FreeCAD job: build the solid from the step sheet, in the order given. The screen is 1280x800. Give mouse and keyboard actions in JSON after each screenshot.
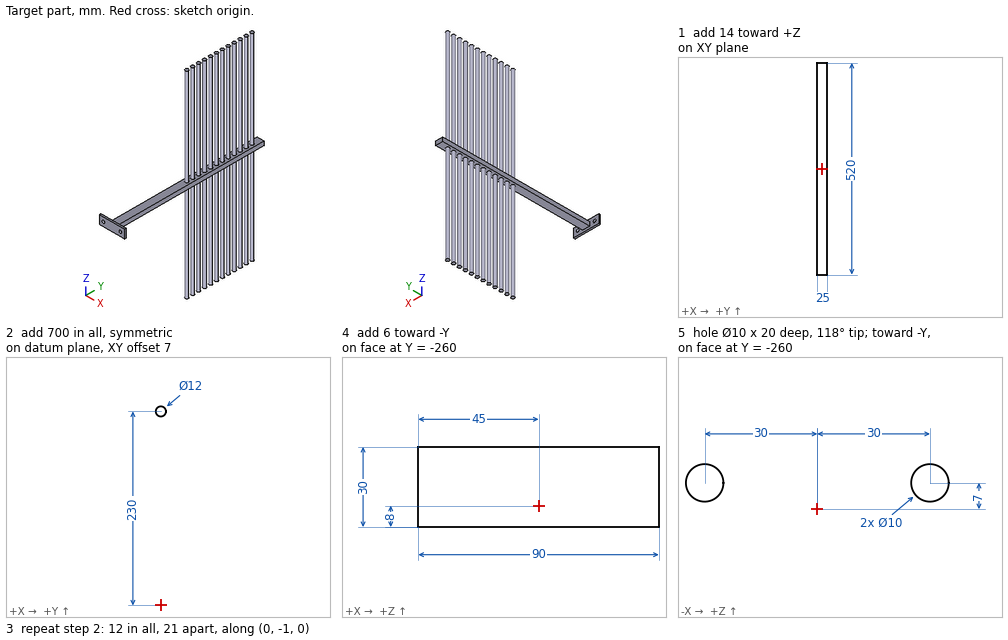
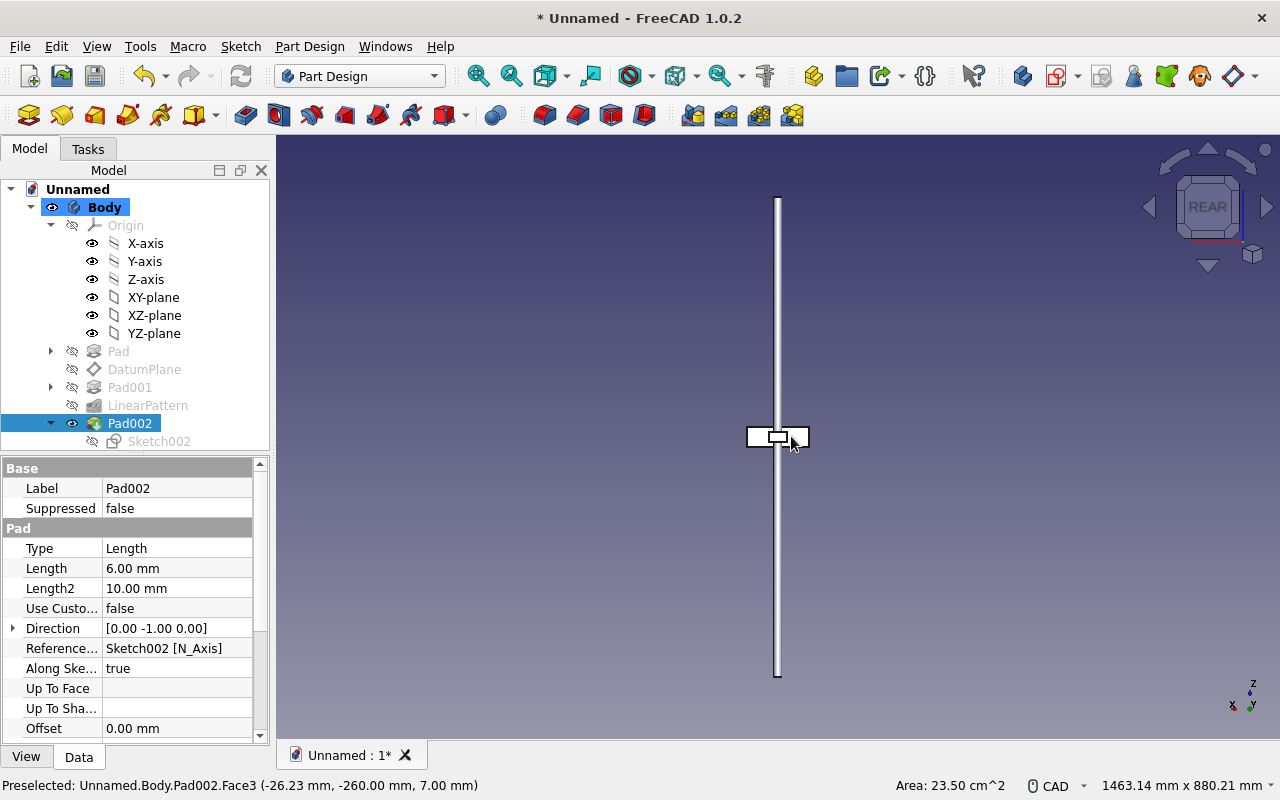
{"action": "left_click", "coordinate": [1056, 76]}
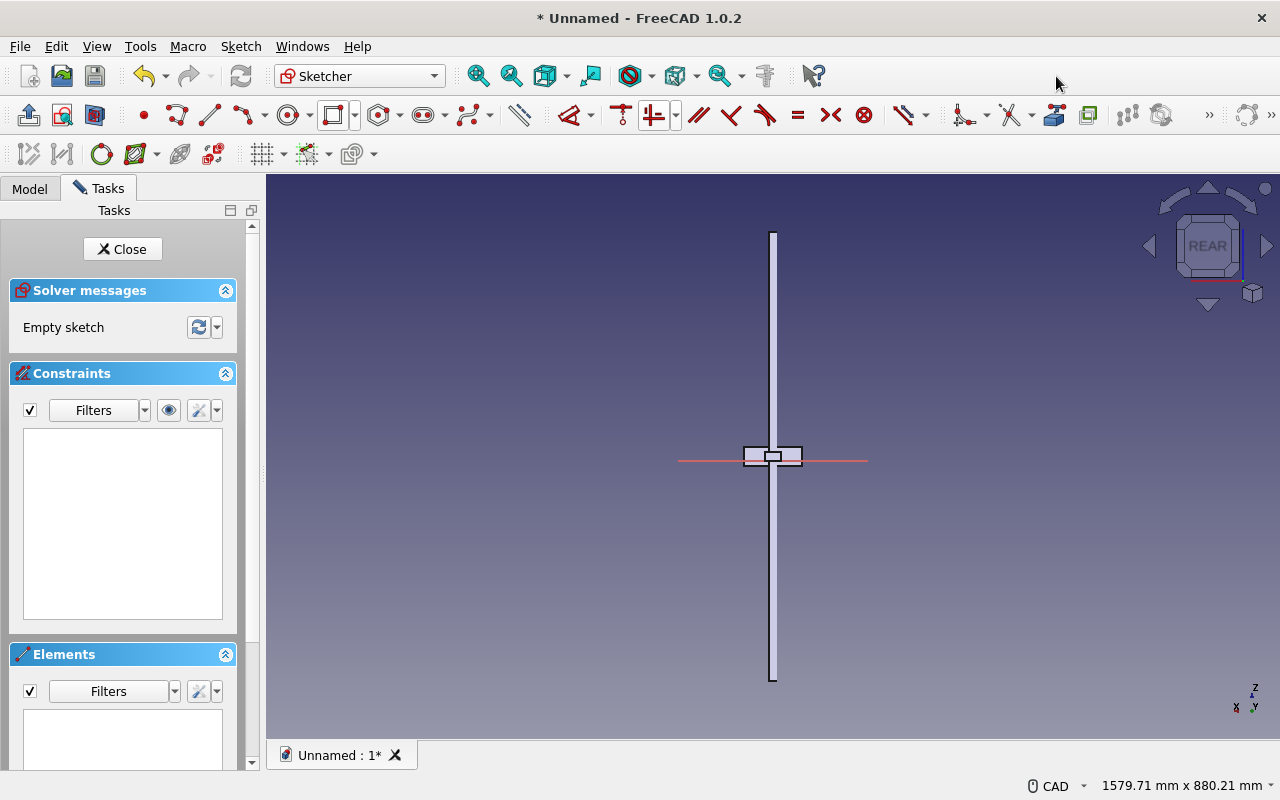
{"action": "left_click", "coordinate": [95, 116]}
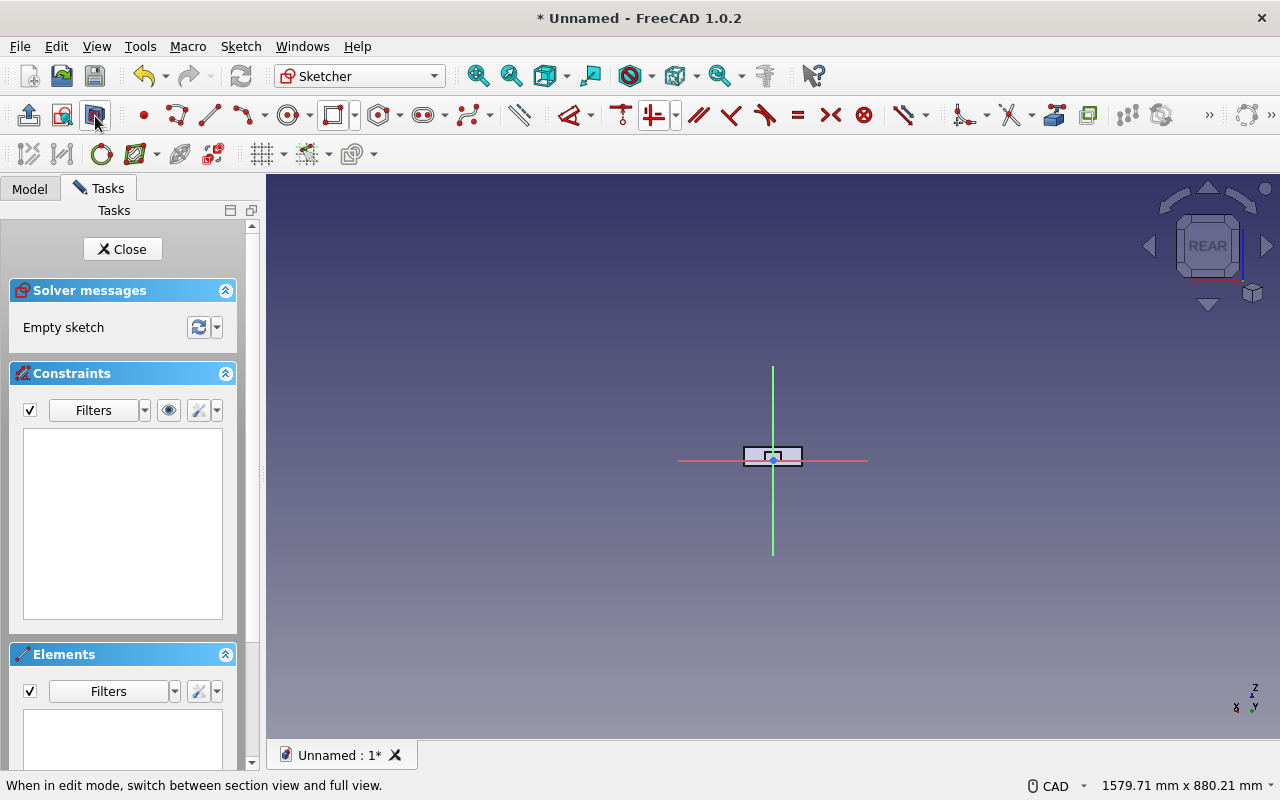
{"action": "scroll", "coordinate": [778, 457], "scroll_direction": "up", "scroll_amount": 13}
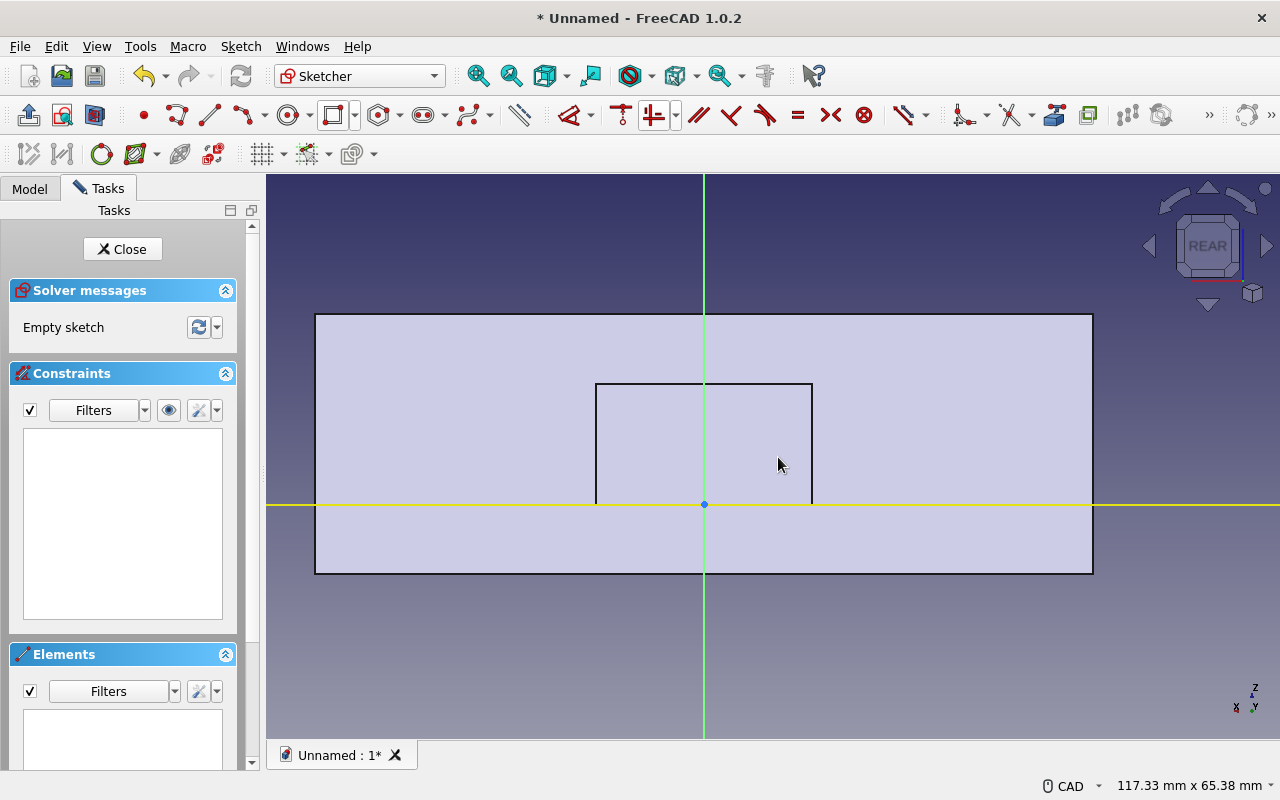
{"action": "left_click", "coordinate": [288, 116]}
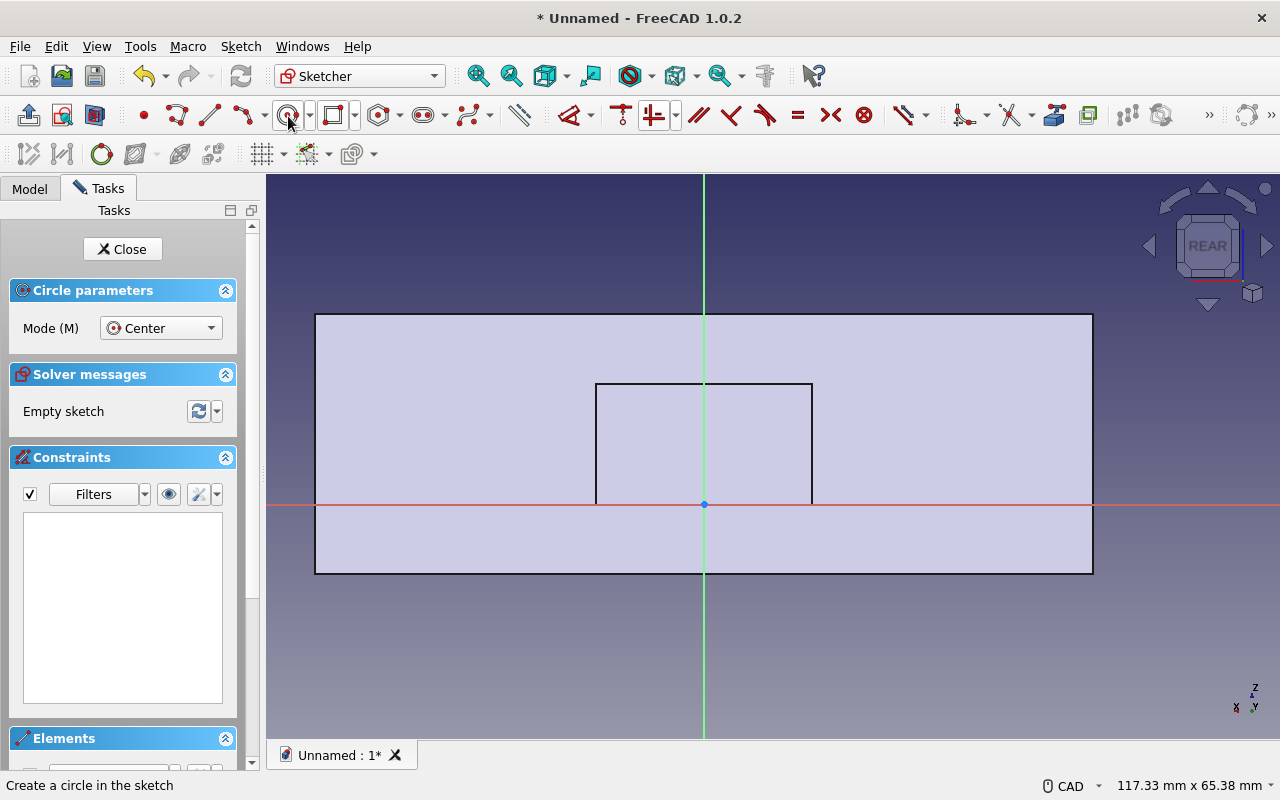
{"action": "left_click", "coordinate": [964, 444]}
{"action": "left_click", "coordinate": [994, 413]}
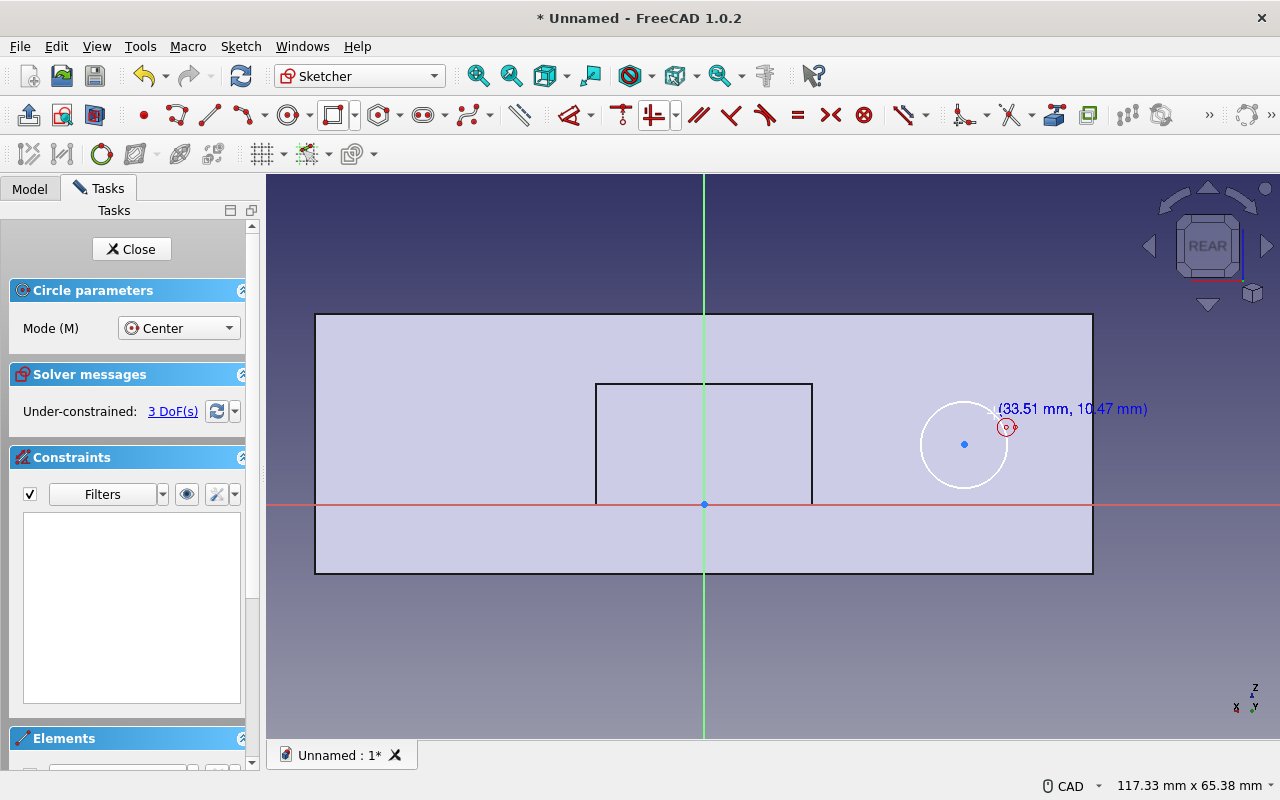
{"action": "left_click", "coordinate": [445, 444]}
{"action": "left_click", "coordinate": [476, 413]}
{"action": "key", "text": "Escape"}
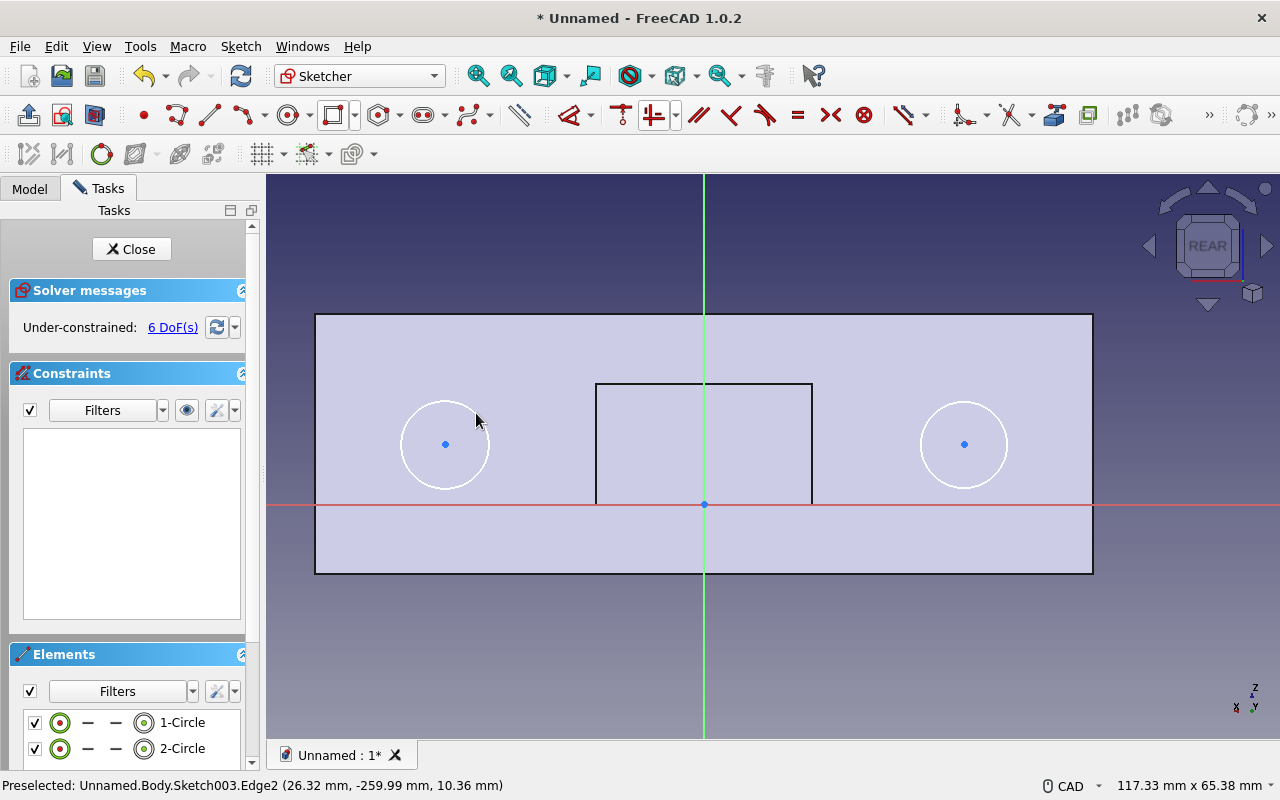
{"action": "left_click", "coordinate": [994, 414]}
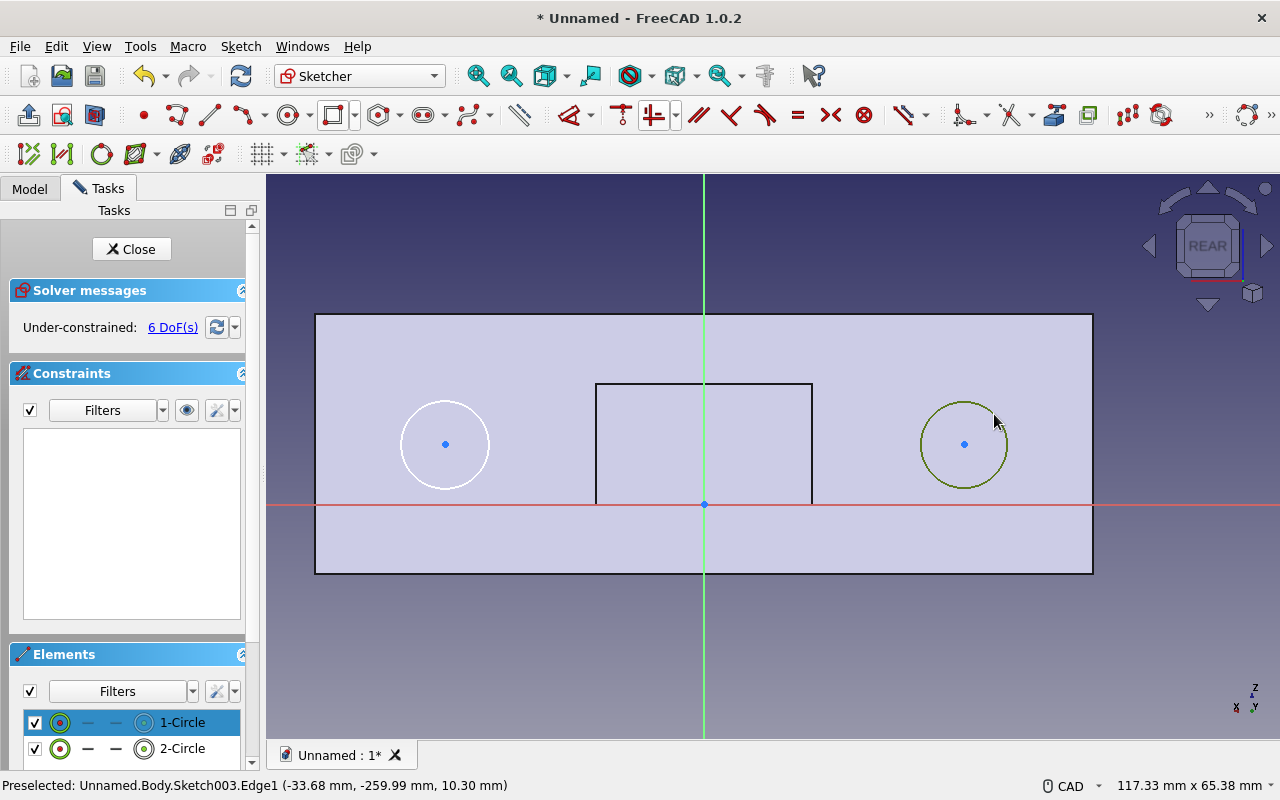
{"action": "left_click", "coordinate": [476, 414]}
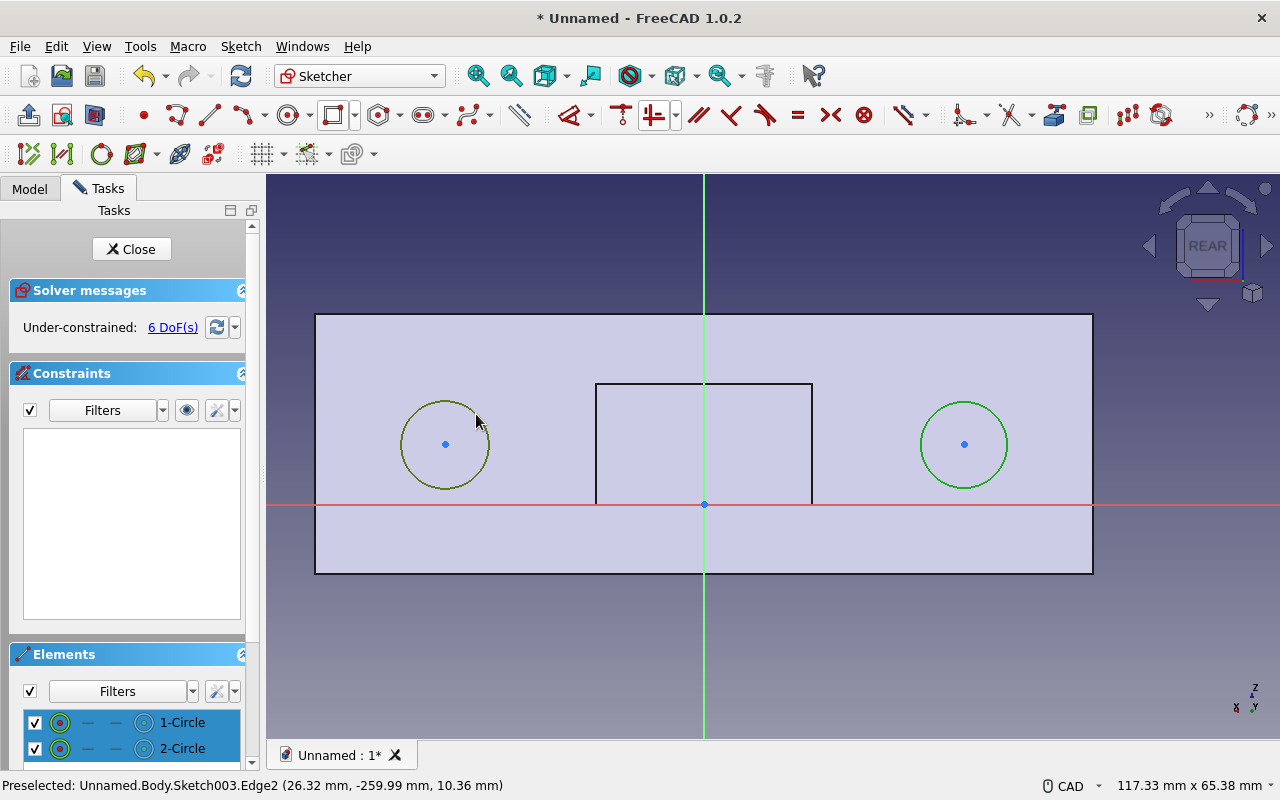
{"action": "left_click", "coordinate": [798, 116]}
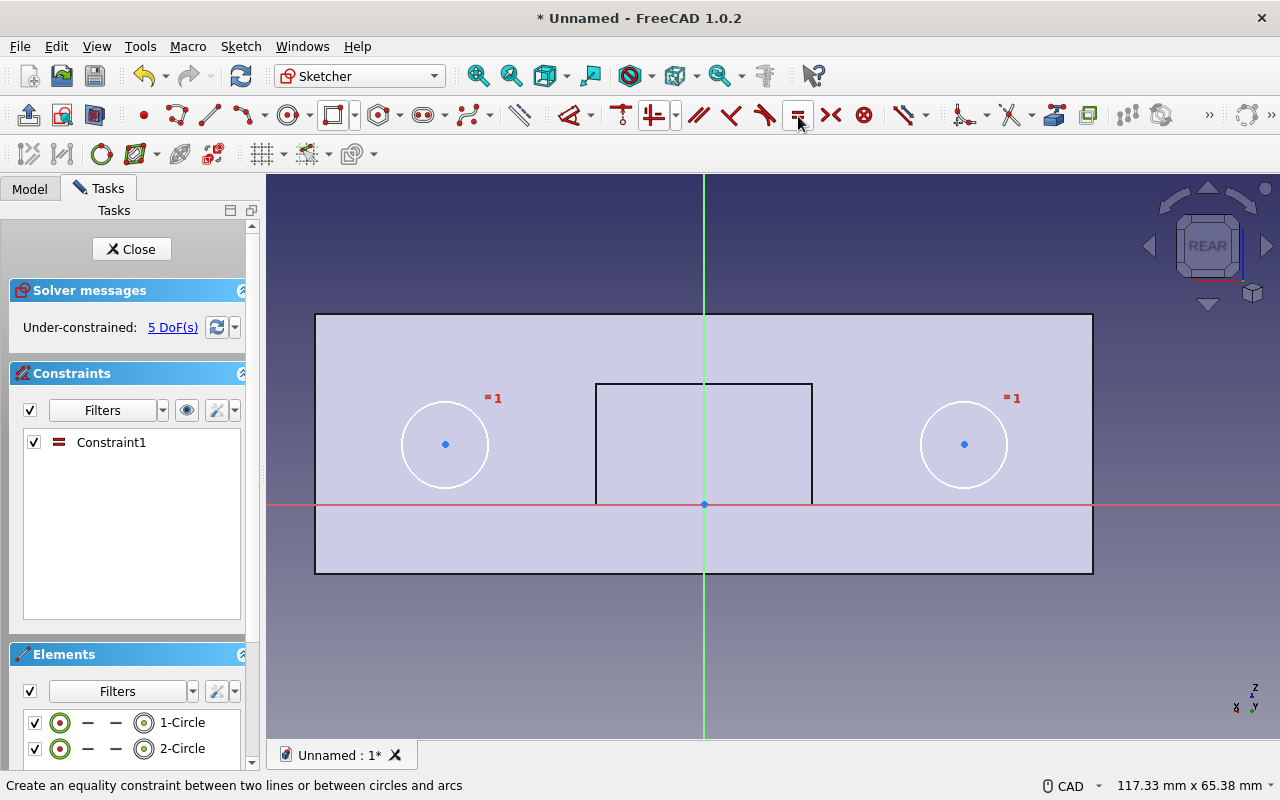
{"action": "left_click", "coordinate": [964, 445]}